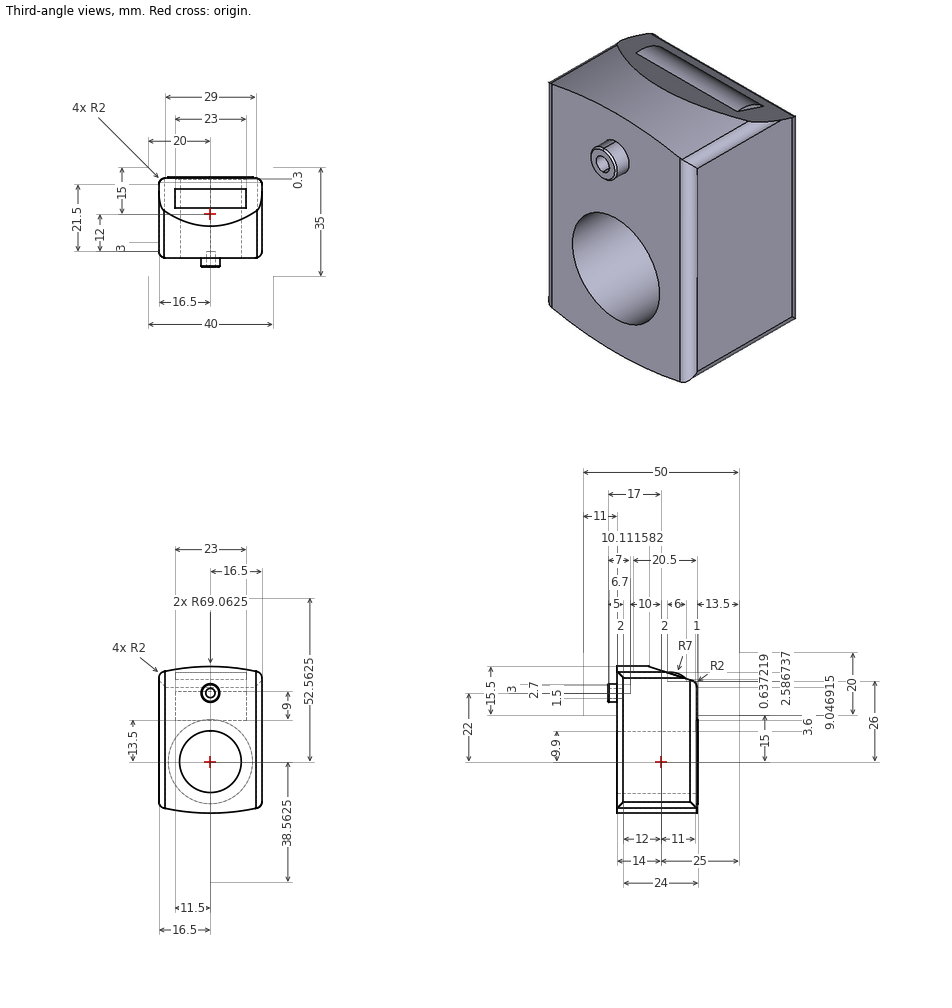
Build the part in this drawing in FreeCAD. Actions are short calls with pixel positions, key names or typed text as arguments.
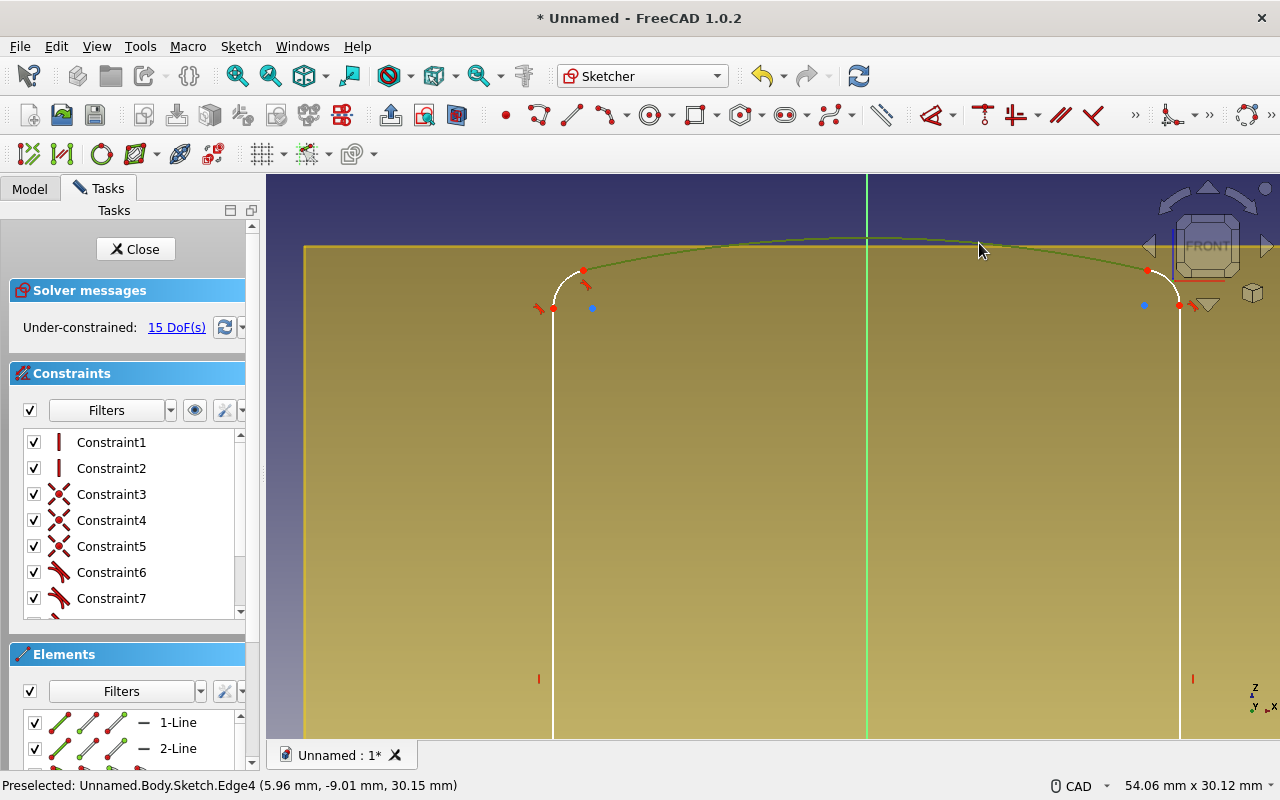
scroll(572, 276, down, 4)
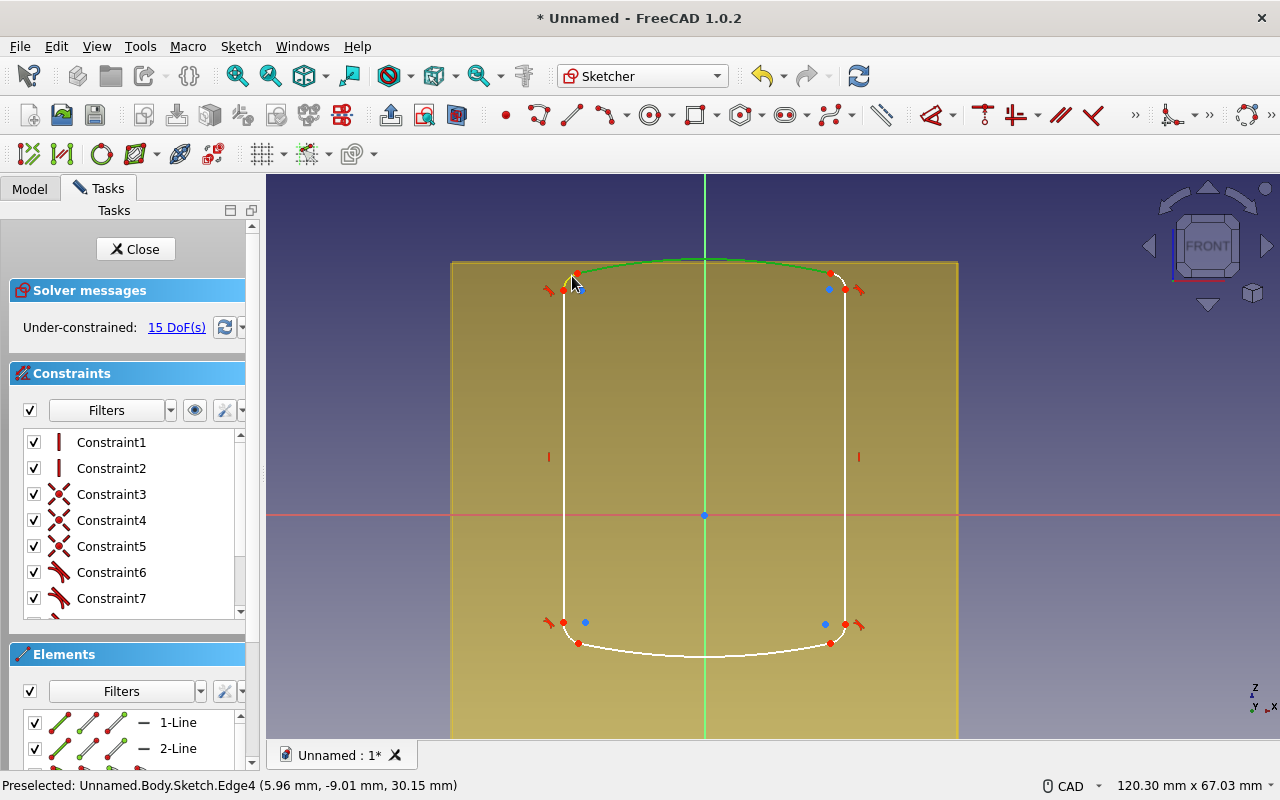
scroll(844, 282, up, 4)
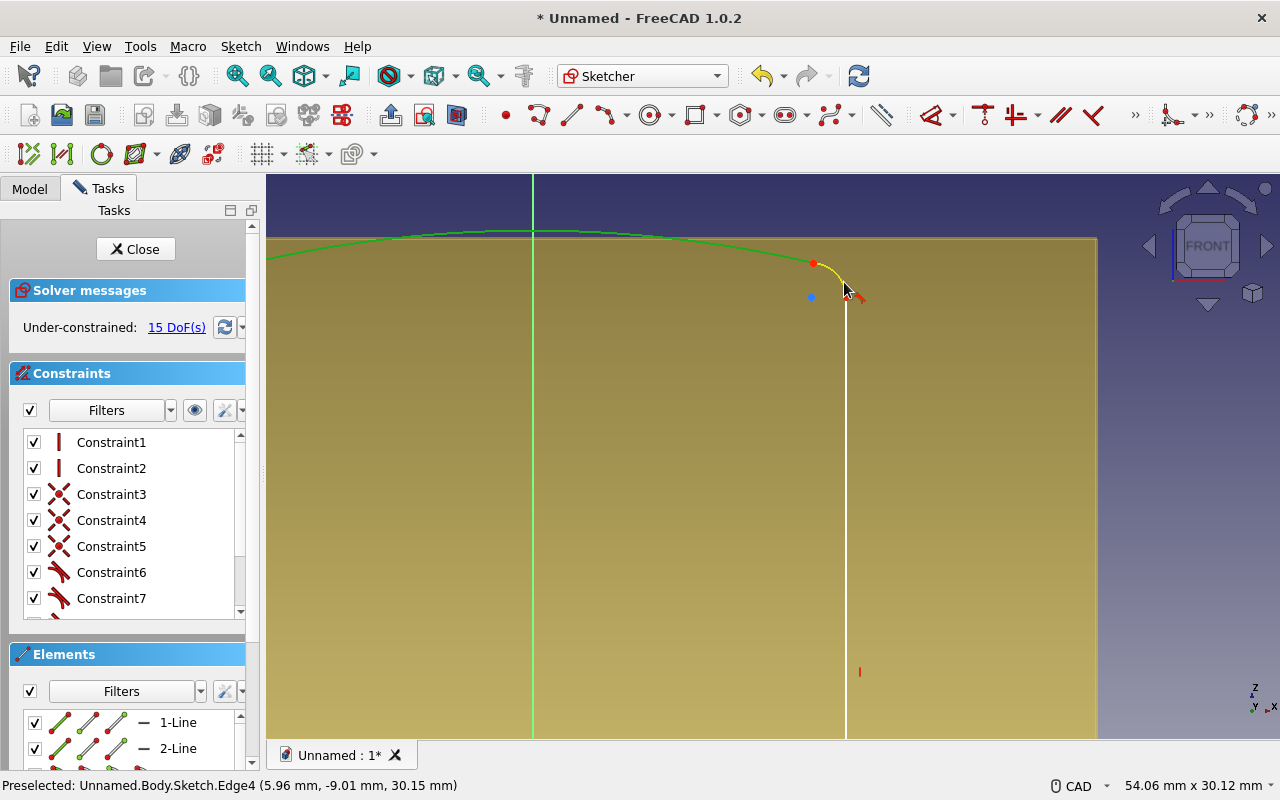
click(843, 283)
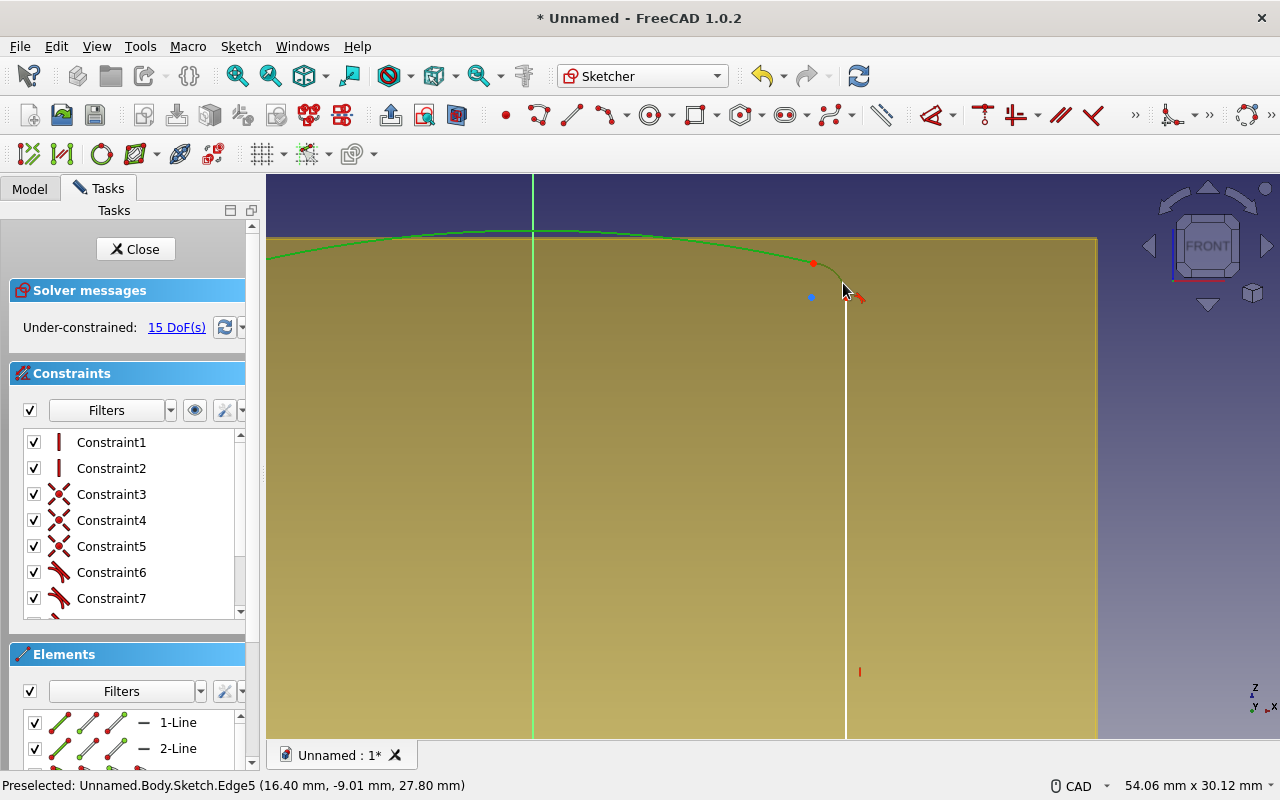
key(t)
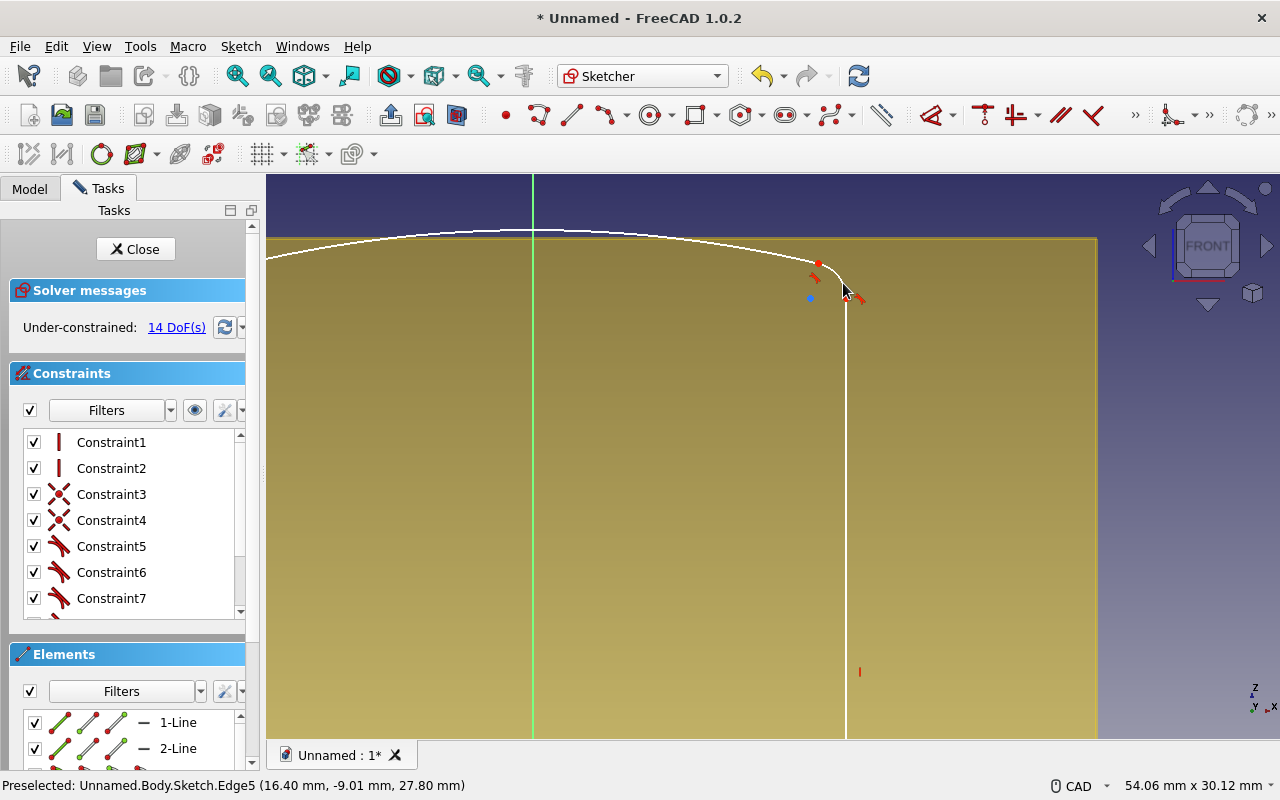
scroll(844, 282, down, 4)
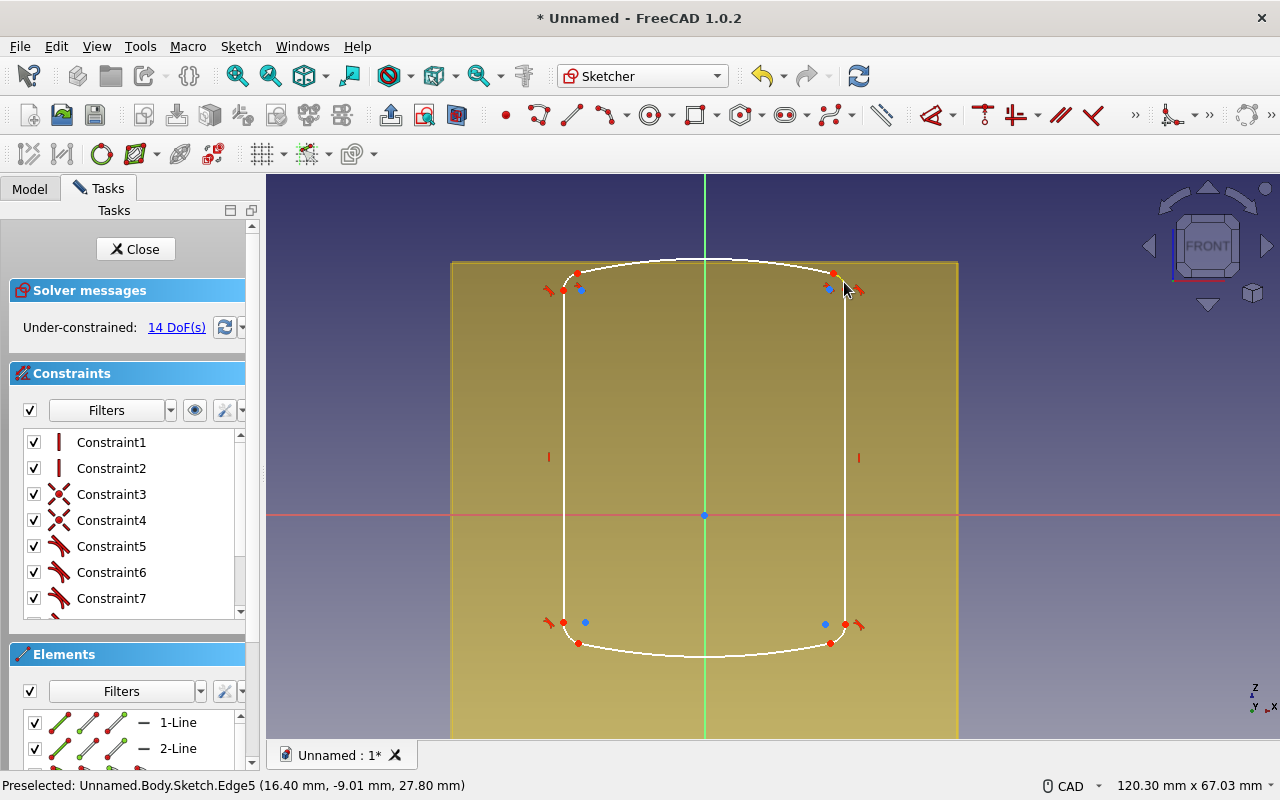
scroll(838, 640, up, 3)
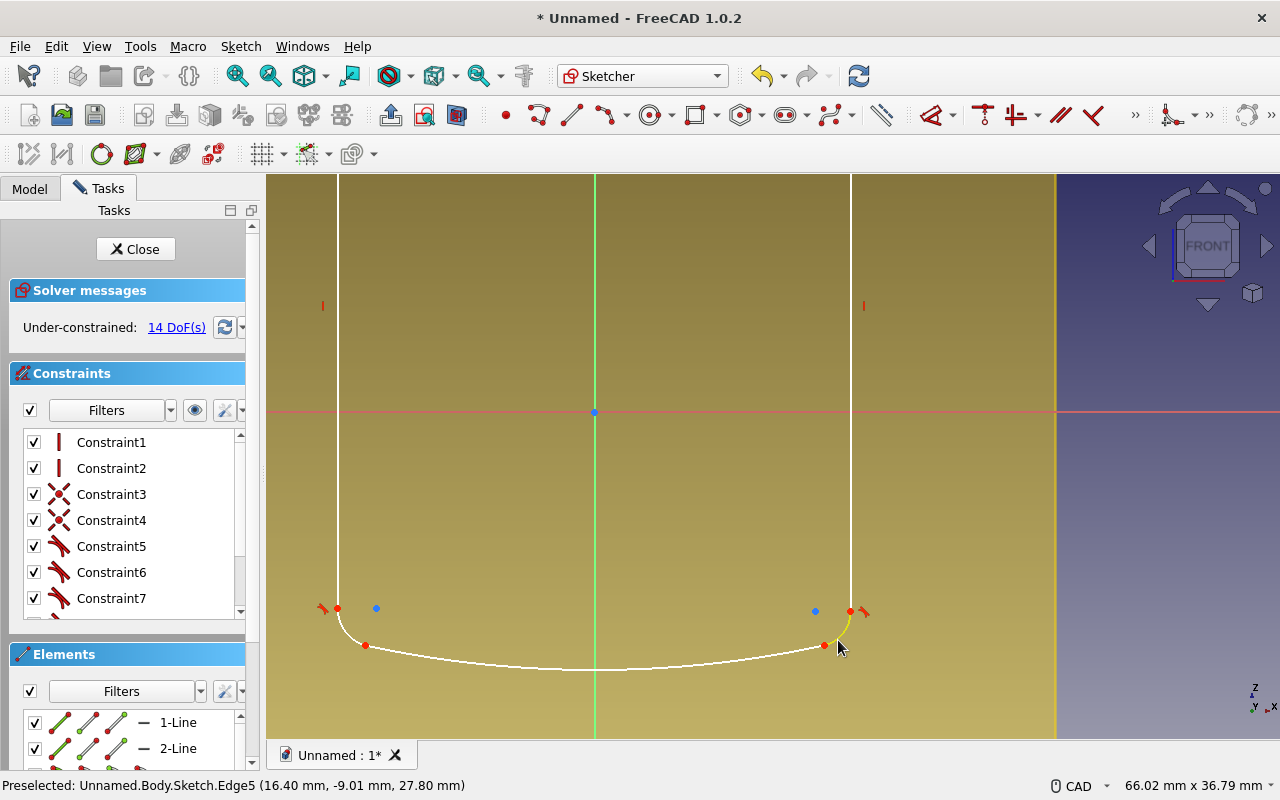
click(837, 639)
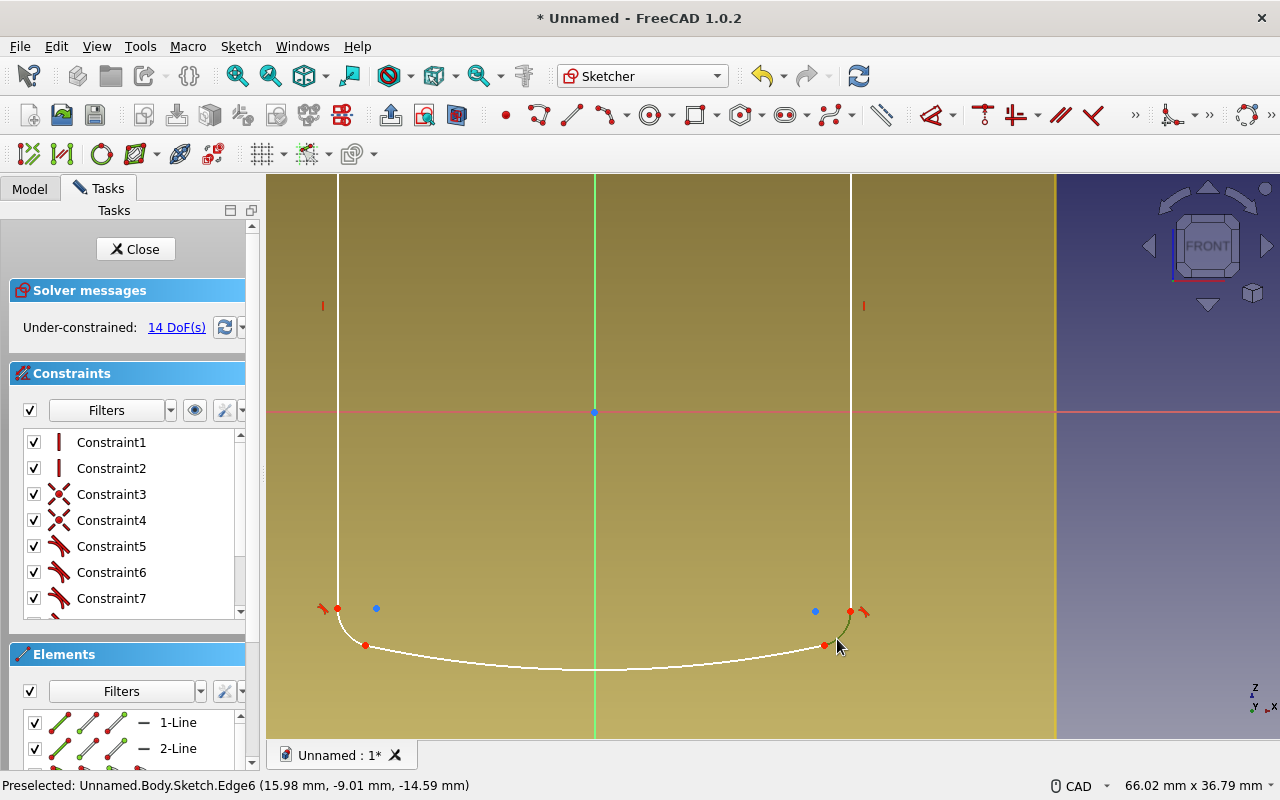
click(502, 666)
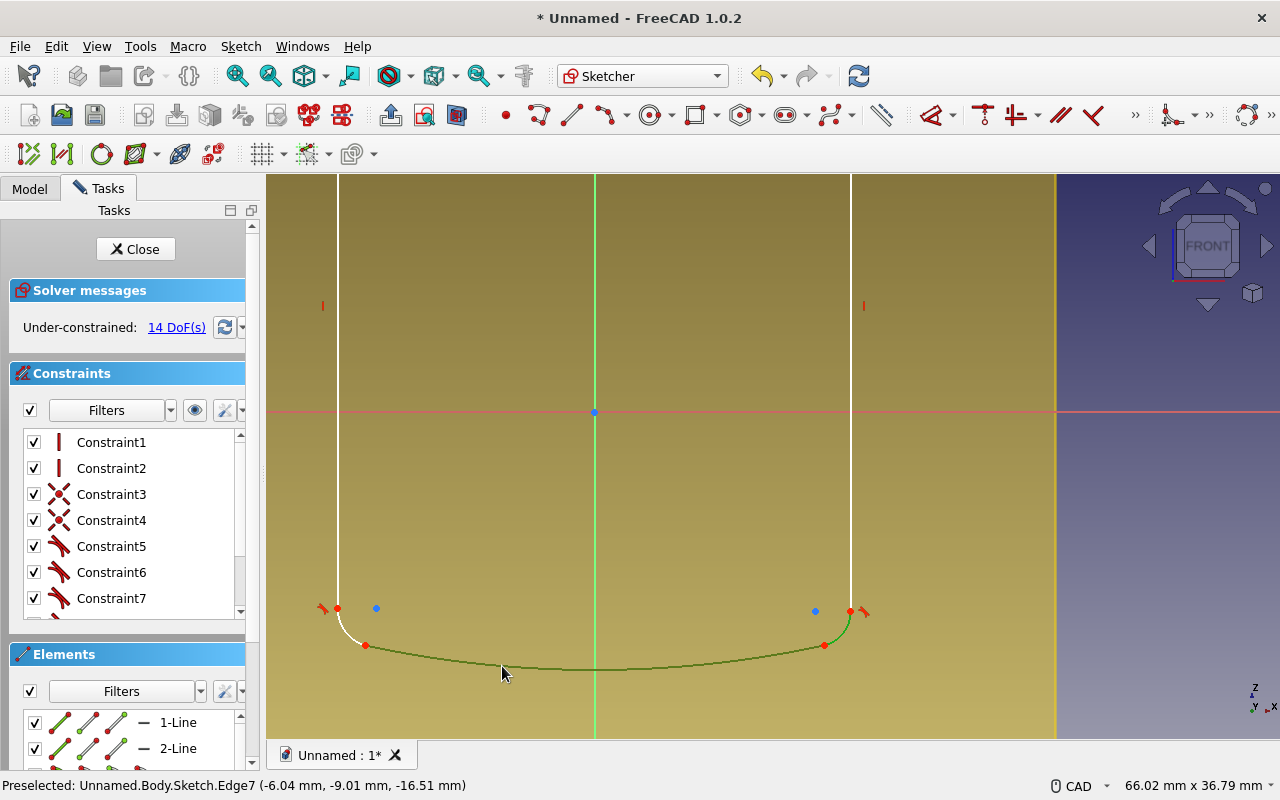
key(t)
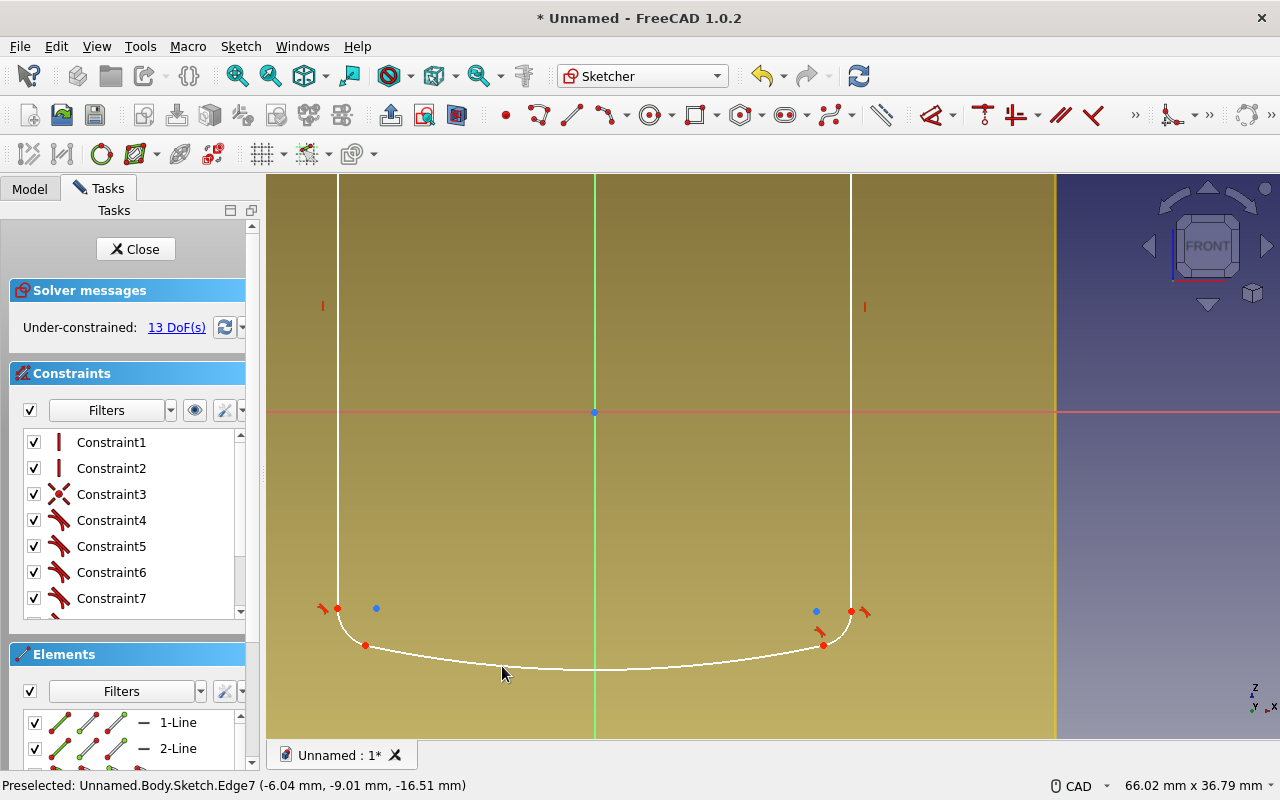
click(502, 666)